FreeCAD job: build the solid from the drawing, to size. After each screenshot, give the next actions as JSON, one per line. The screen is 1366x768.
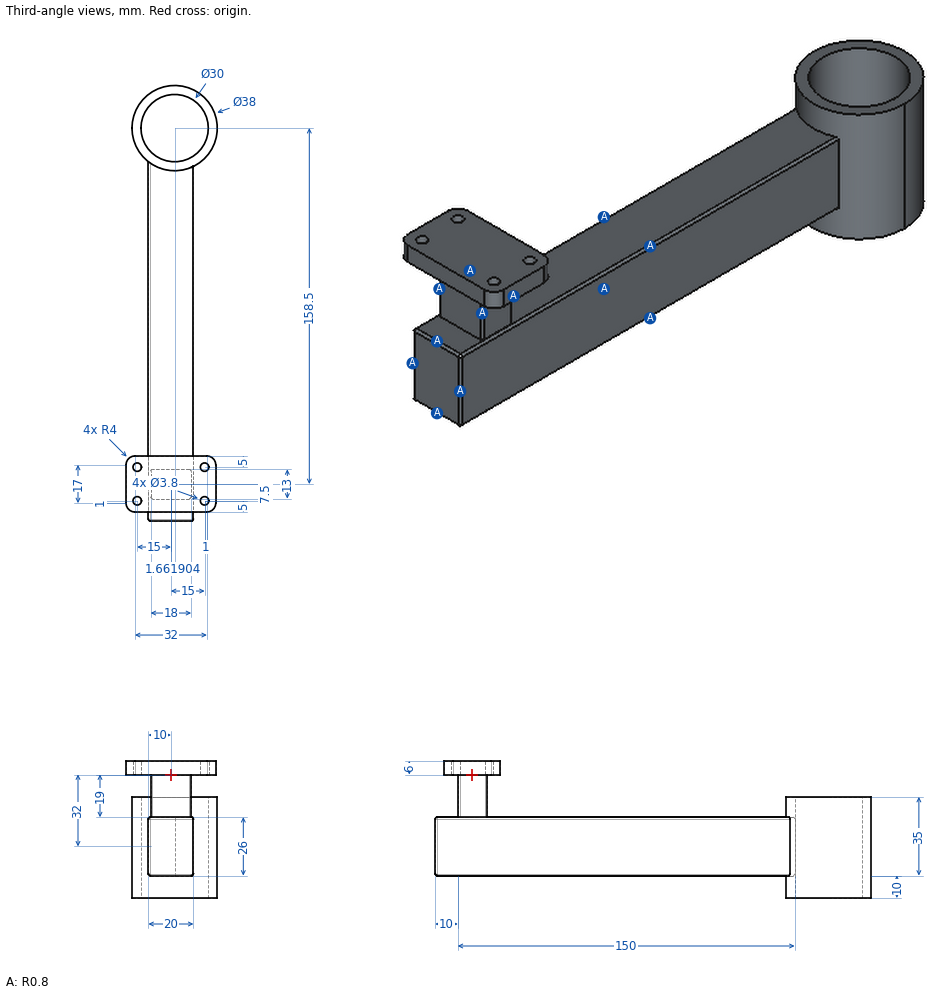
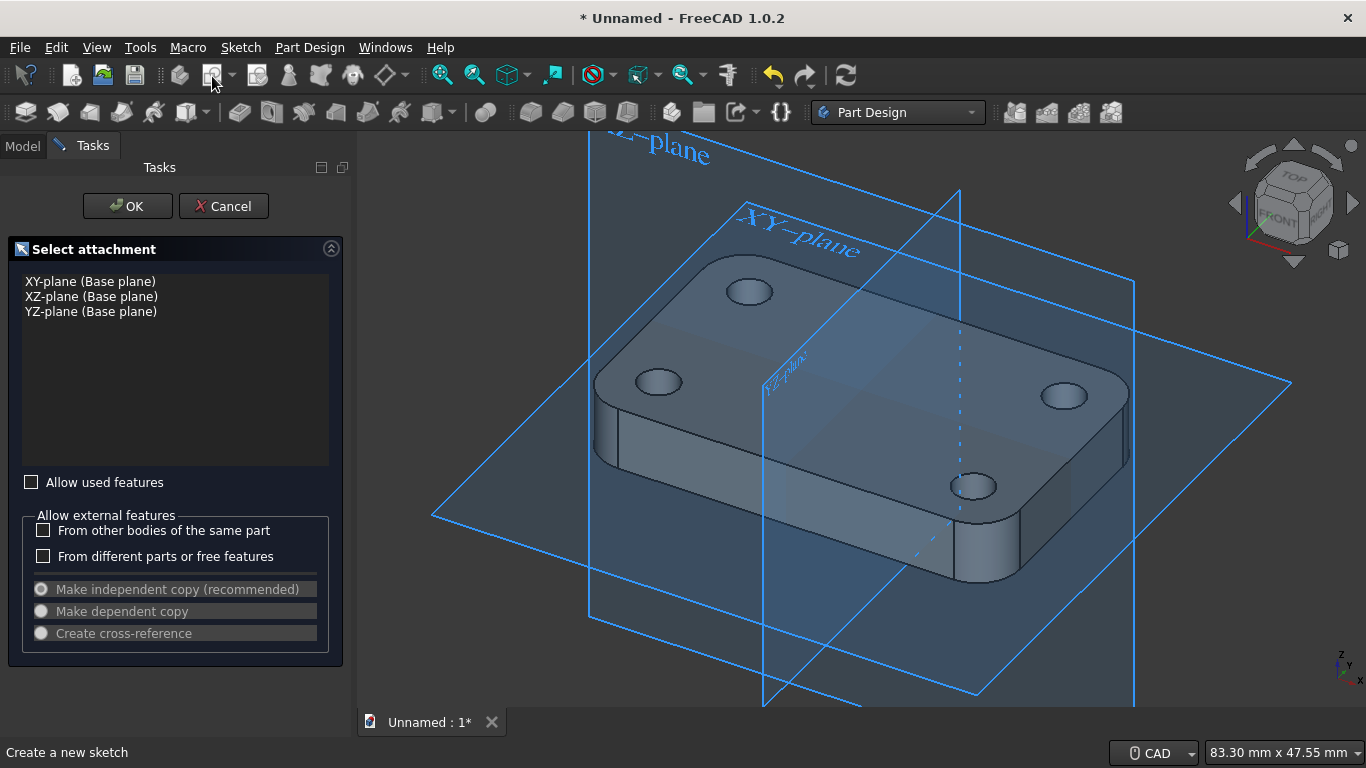
{"action": "left_click", "coordinate": [82, 282]}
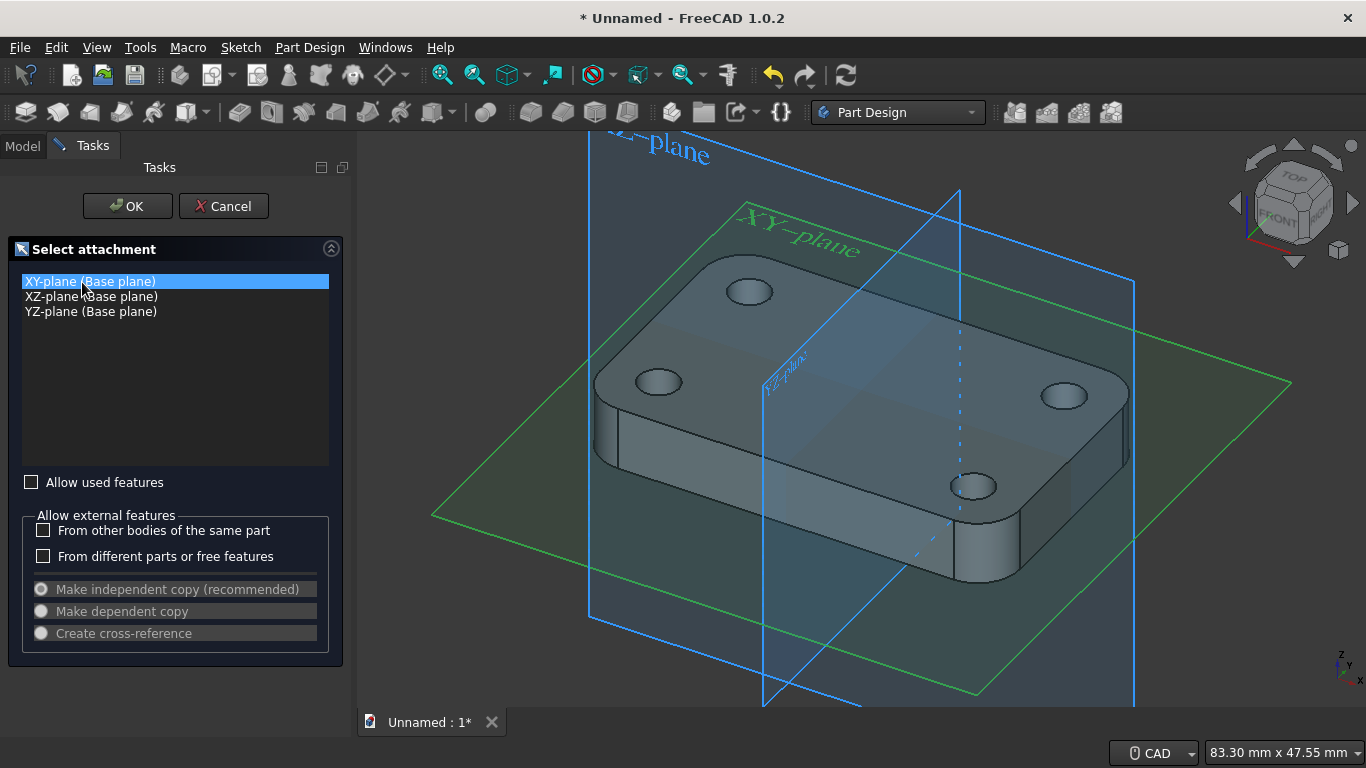
{"action": "left_click", "coordinate": [128, 206]}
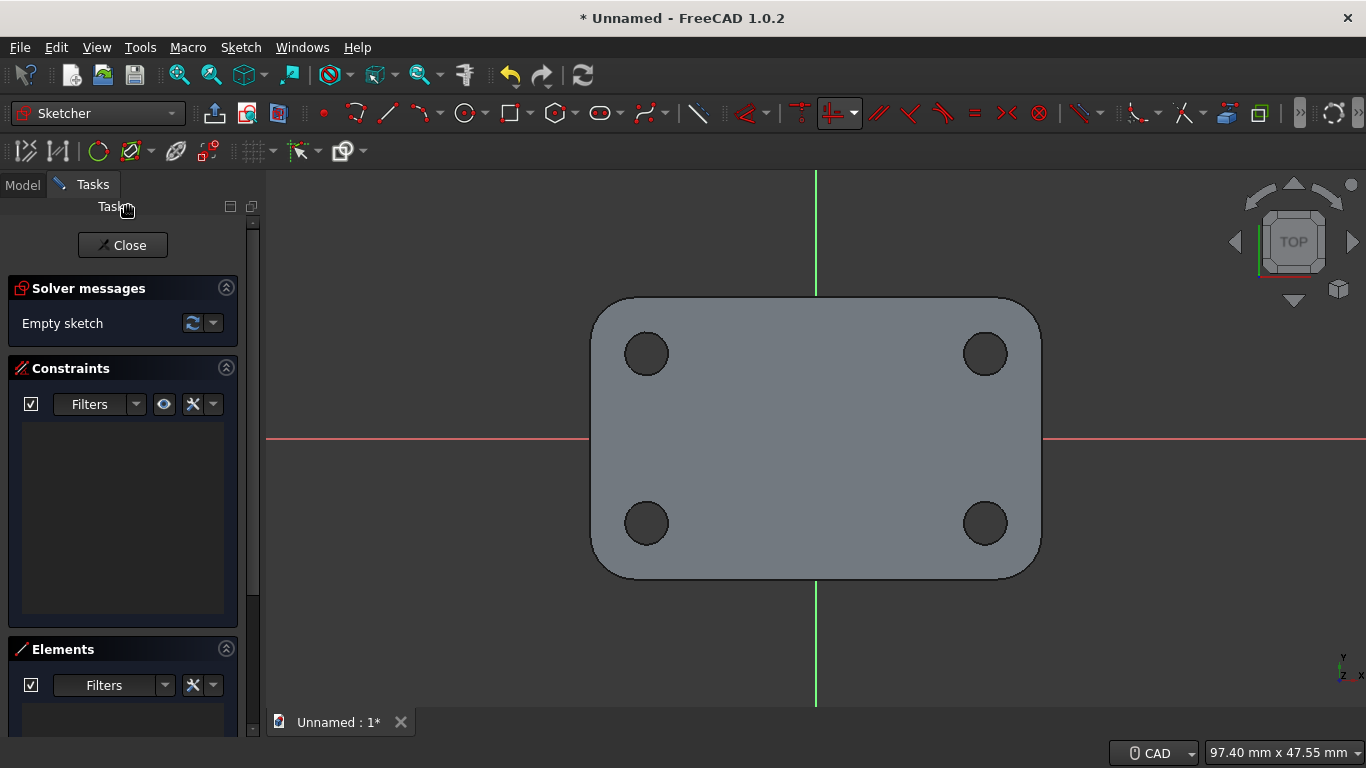
{"action": "key", "text": "q s"}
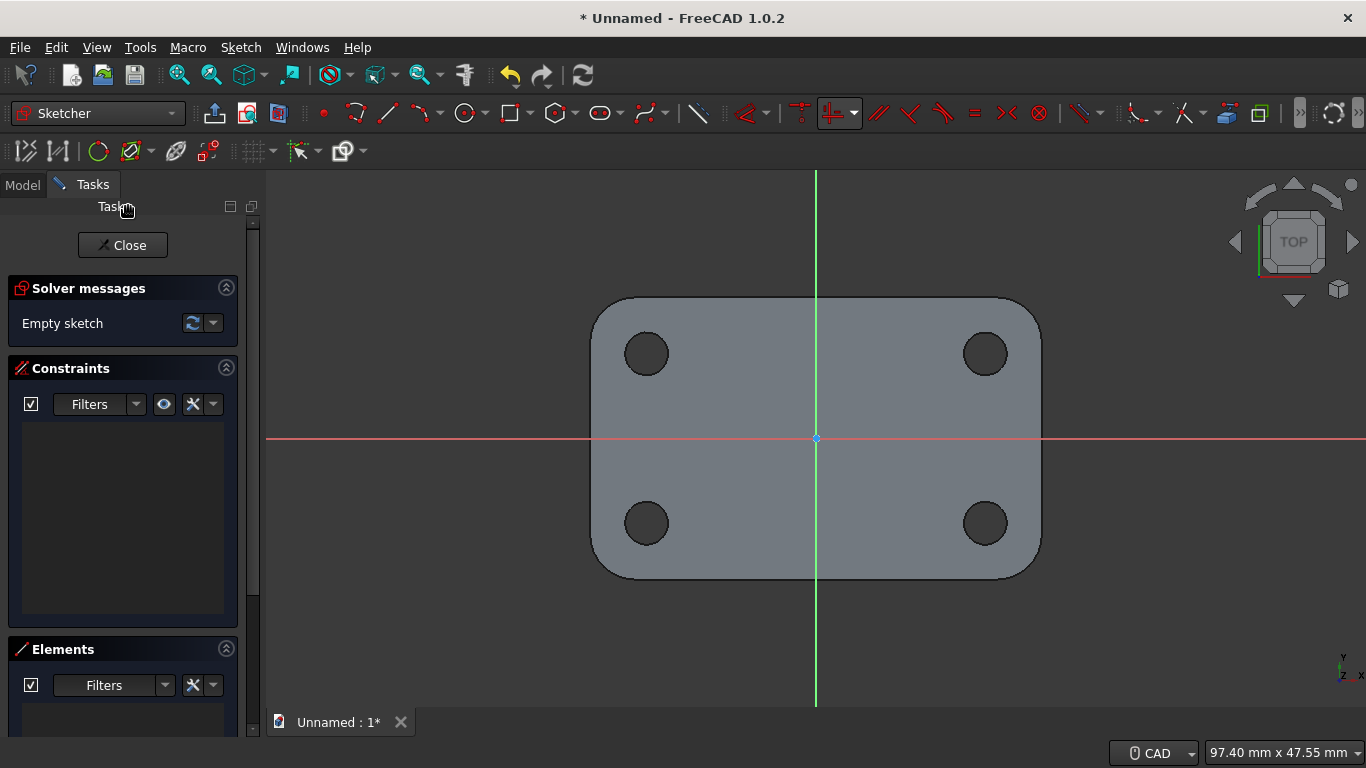
{"action": "scroll", "coordinate": [872, 438], "scroll_direction": "up", "scroll_amount": 4}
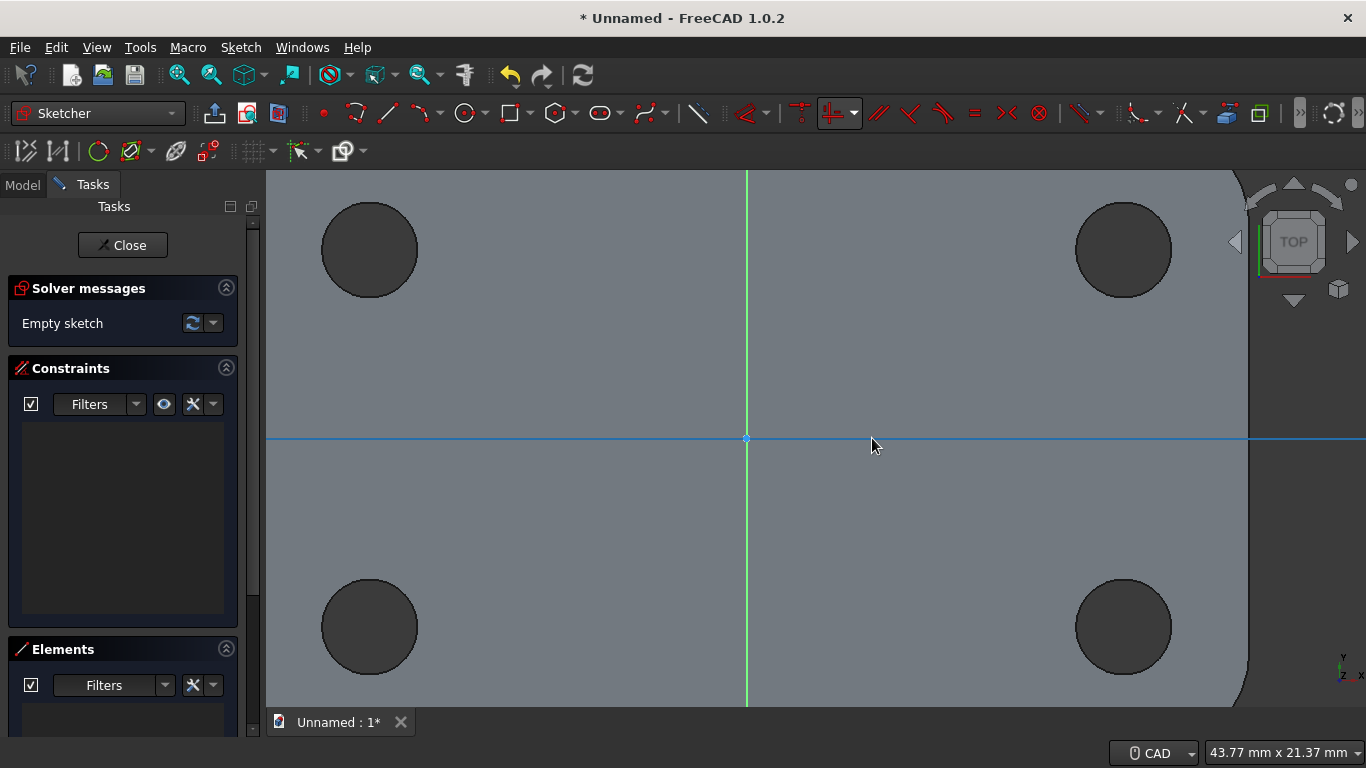
{"action": "left_click", "coordinate": [532, 114]}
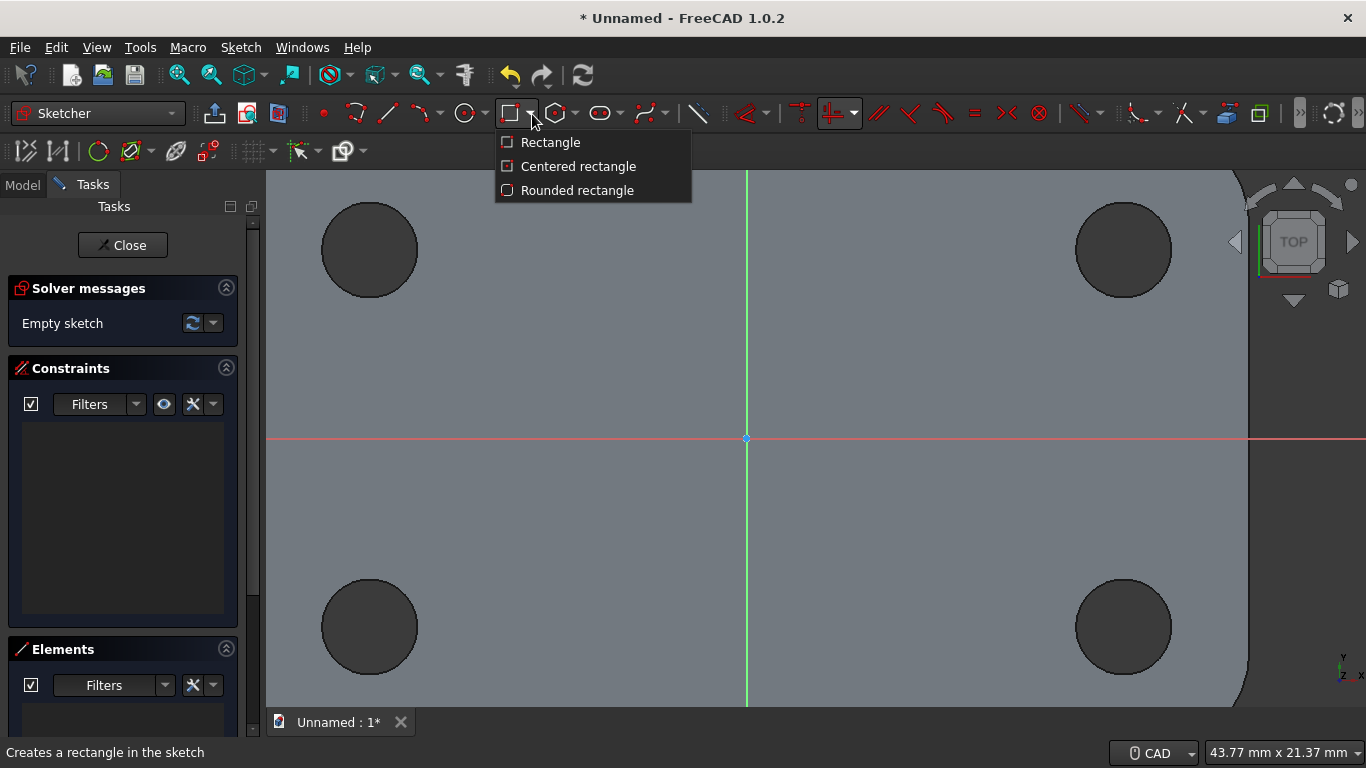
{"action": "left_click", "coordinate": [594, 166]}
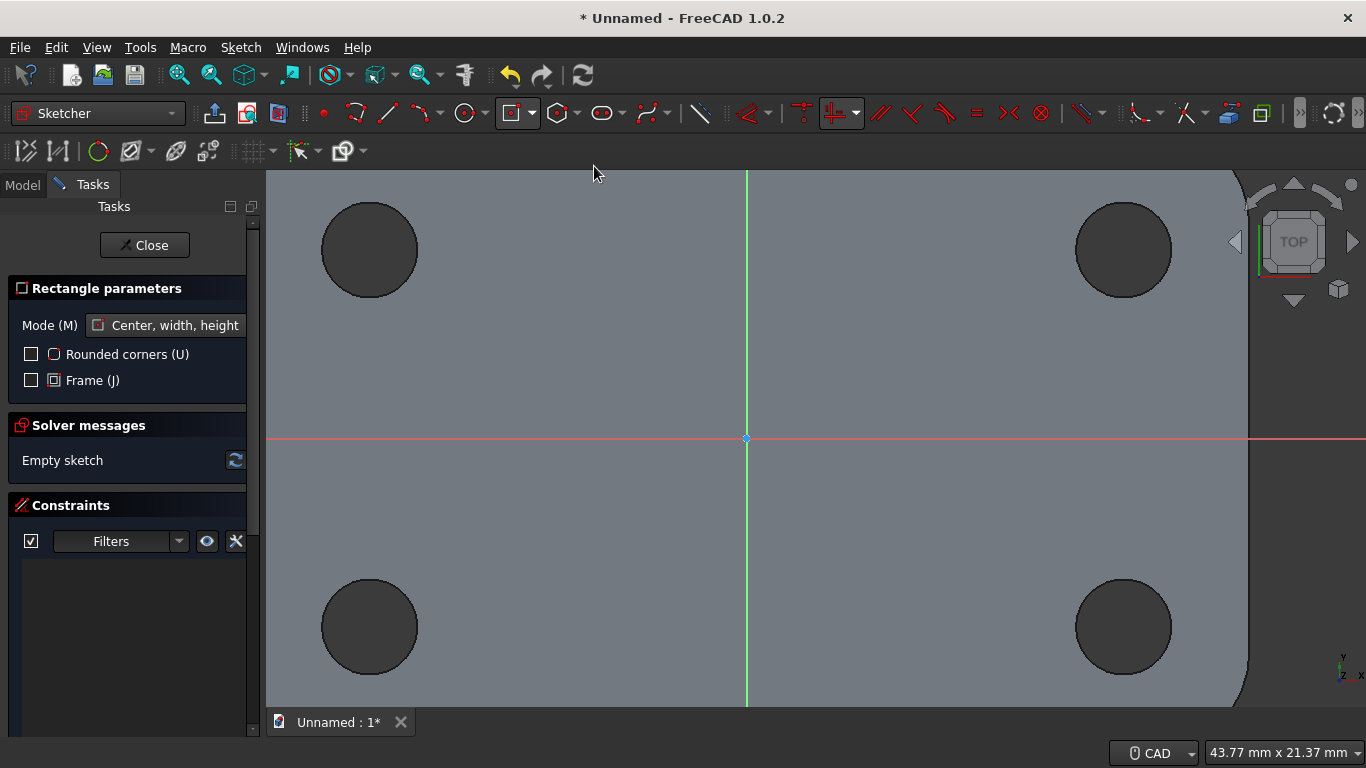
{"action": "left_click", "coordinate": [747, 438]}
{"action": "mouse_move", "coordinate": [973, 275]}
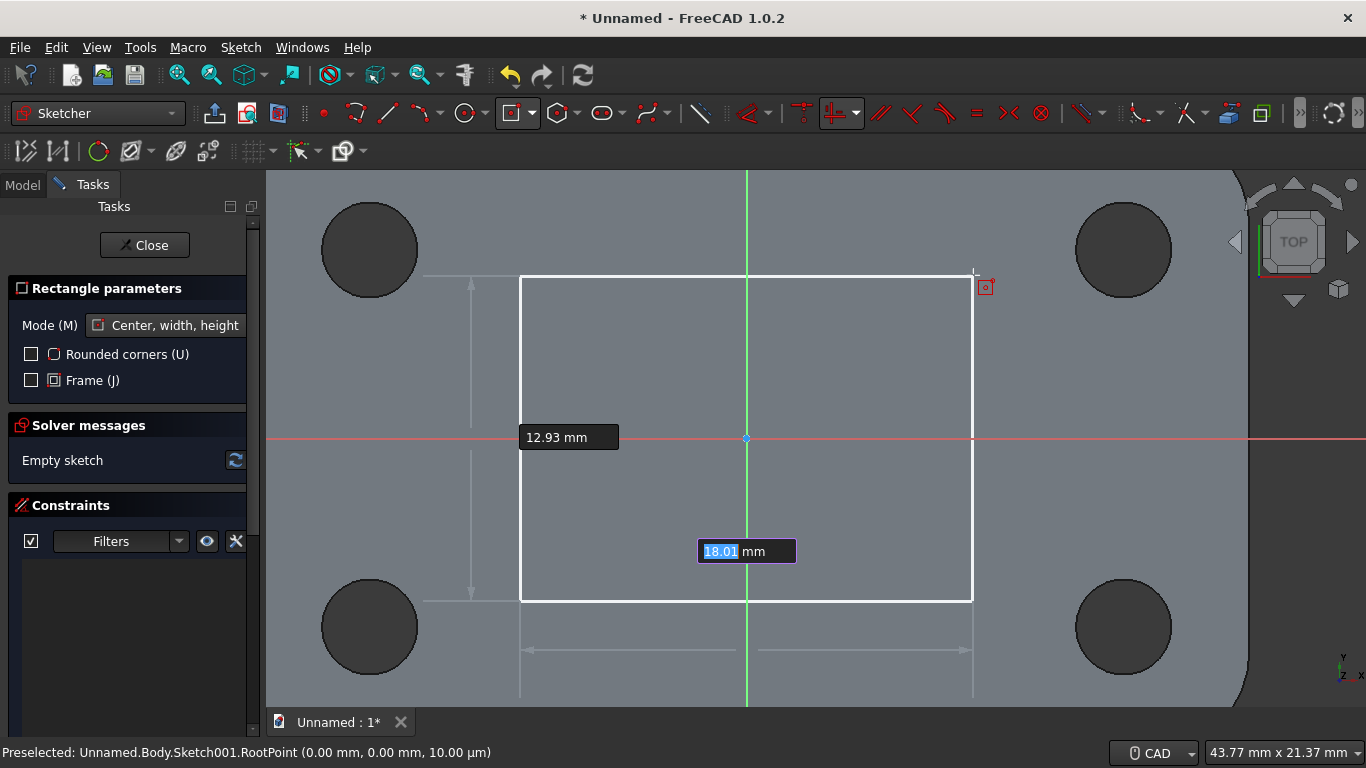
{"action": "type", "text": "18"}
{"action": "key", "text": "Tab"}
{"action": "type", "text": "13"}
{"action": "key", "text": "Return"}
{"action": "key", "text": "Escape"}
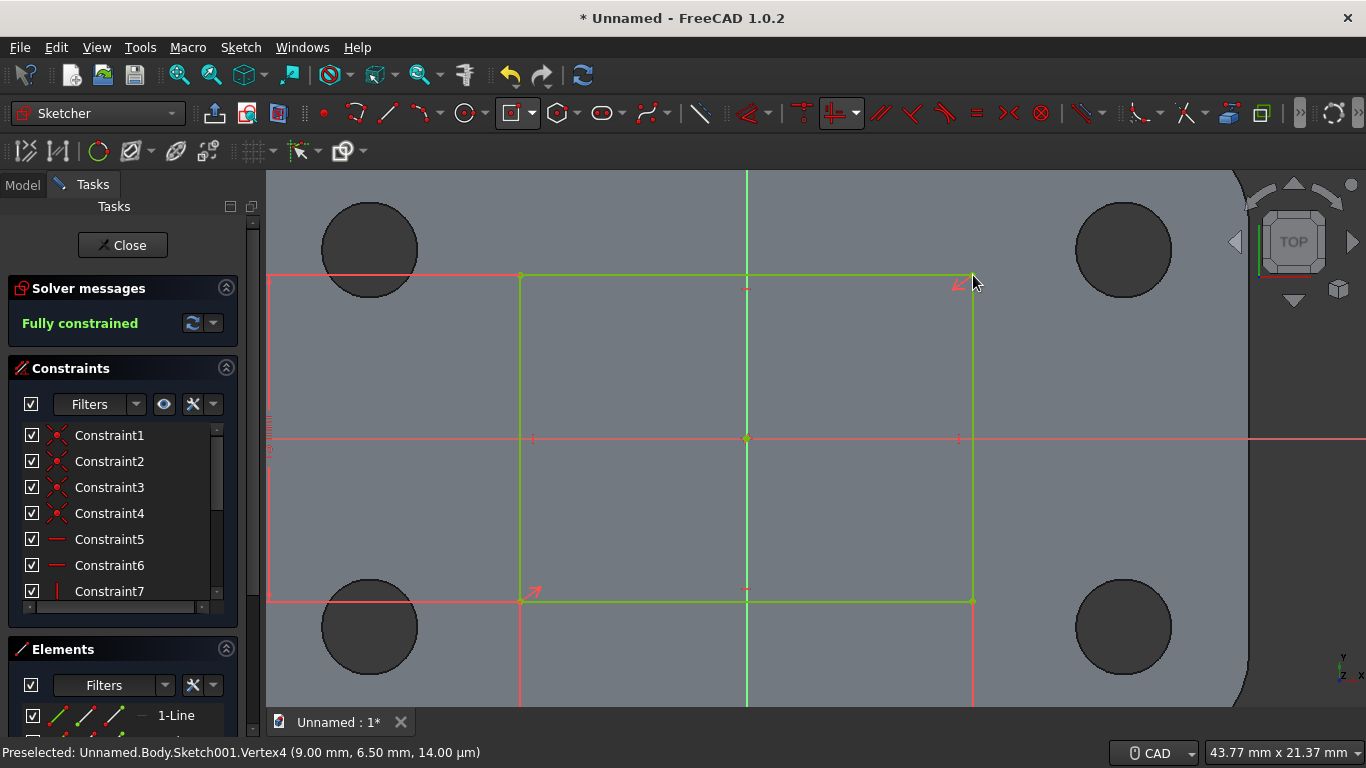
{"action": "left_click", "coordinate": [123, 245]}